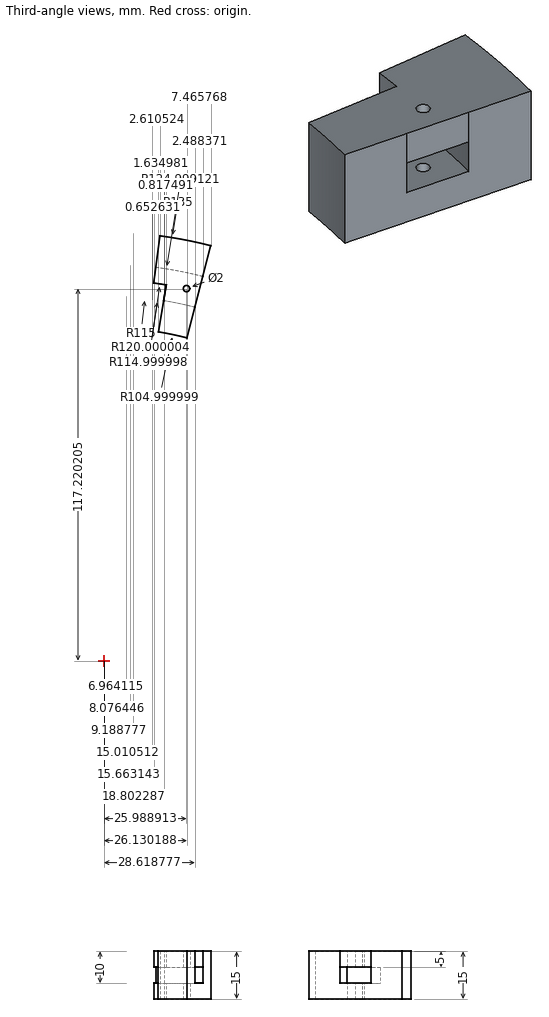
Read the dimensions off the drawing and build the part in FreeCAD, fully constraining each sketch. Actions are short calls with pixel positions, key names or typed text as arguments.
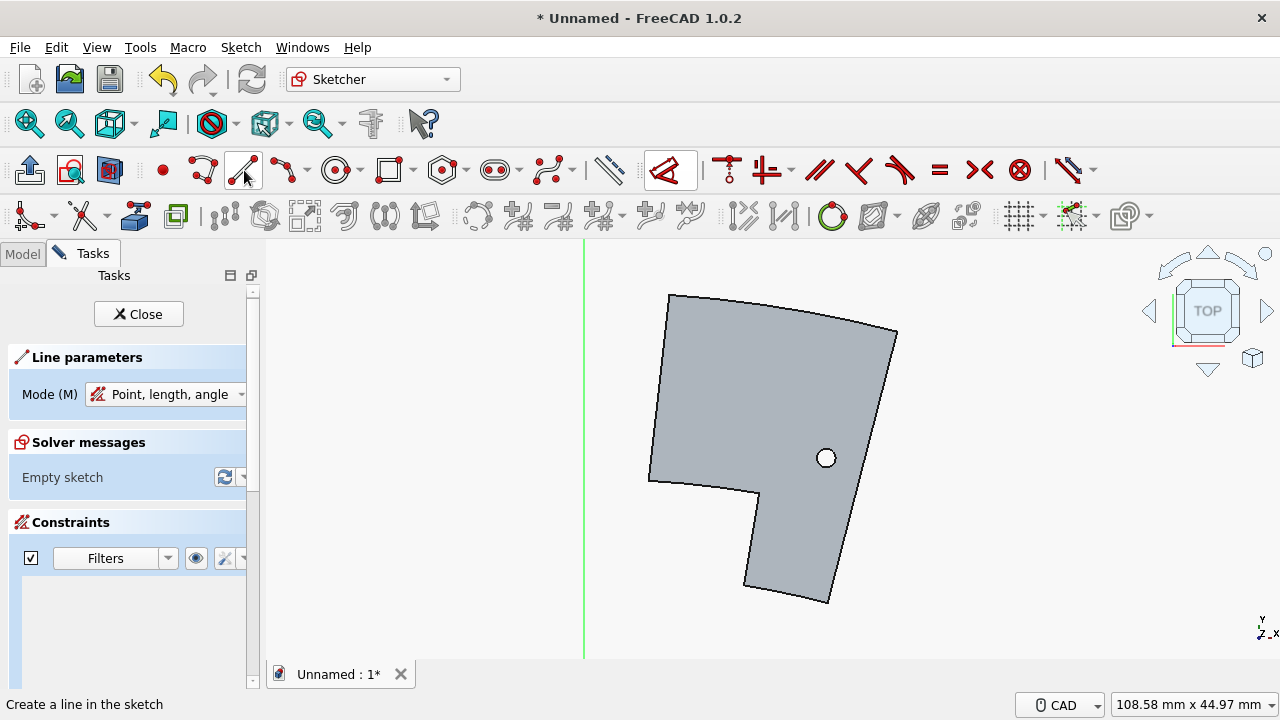
click(584, 292)
click(593, 479)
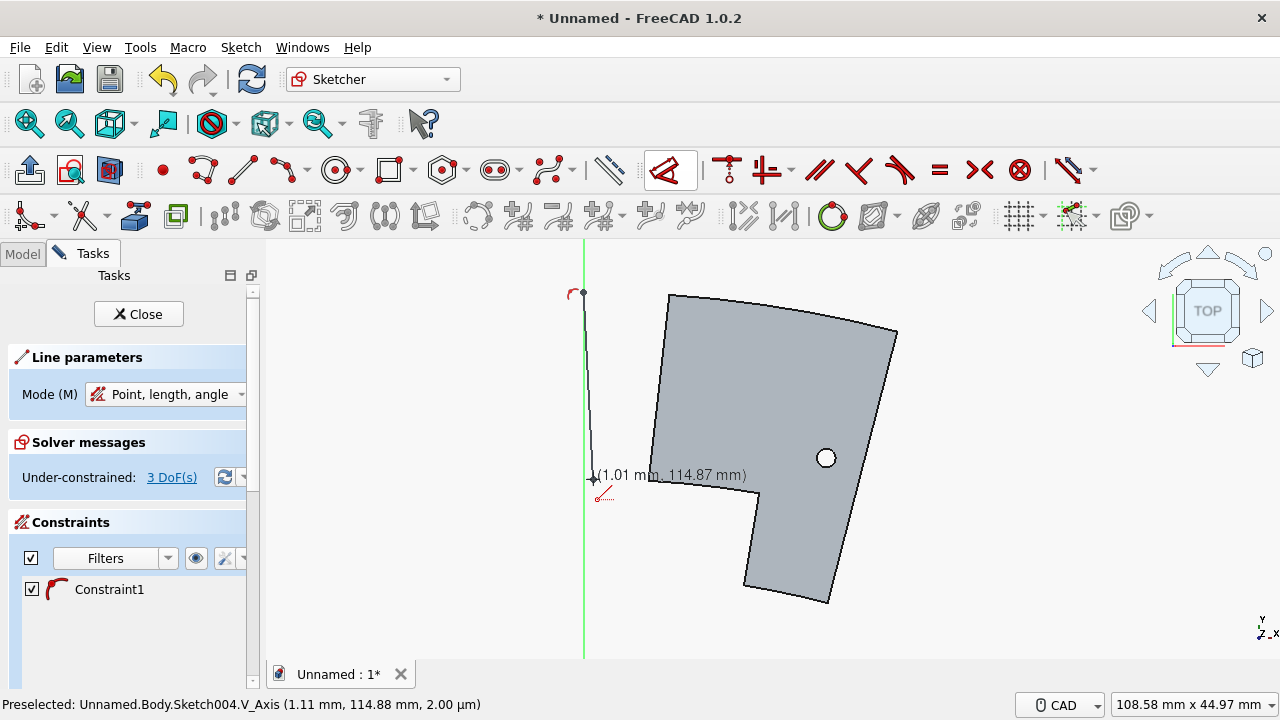
click(724, 488)
click(748, 303)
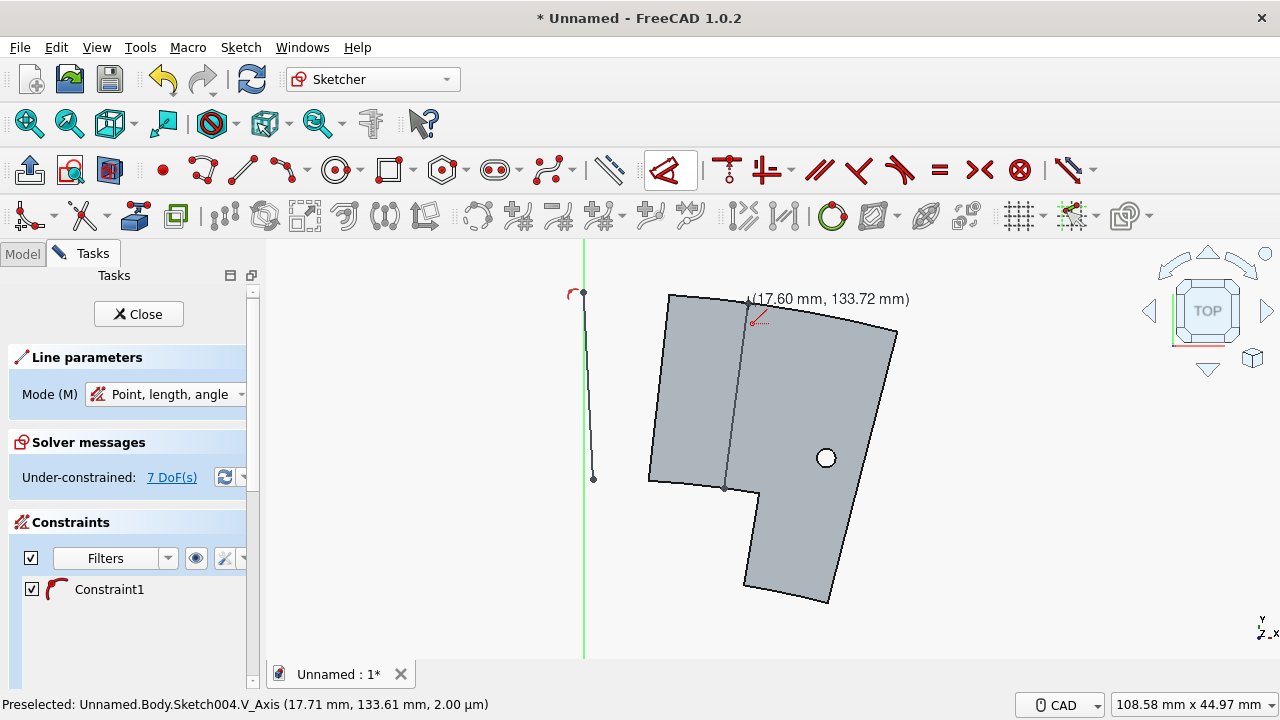
click(284, 170)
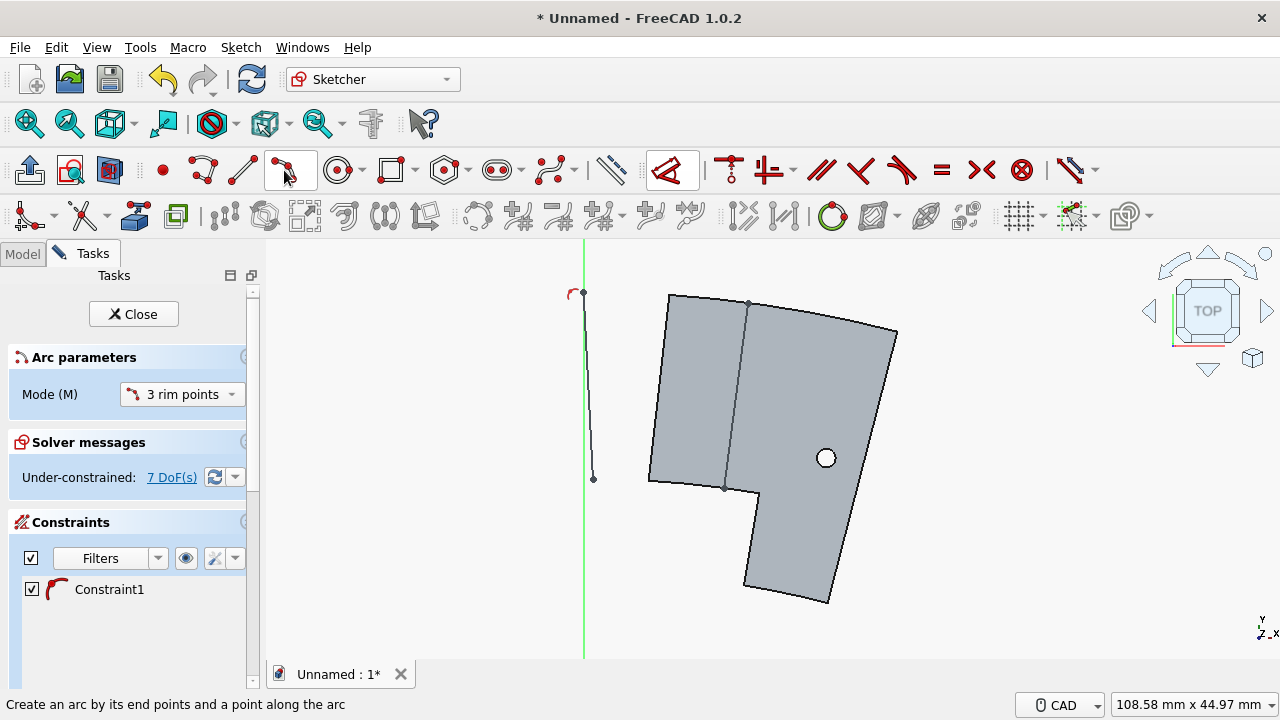
click(593, 480)
click(724, 489)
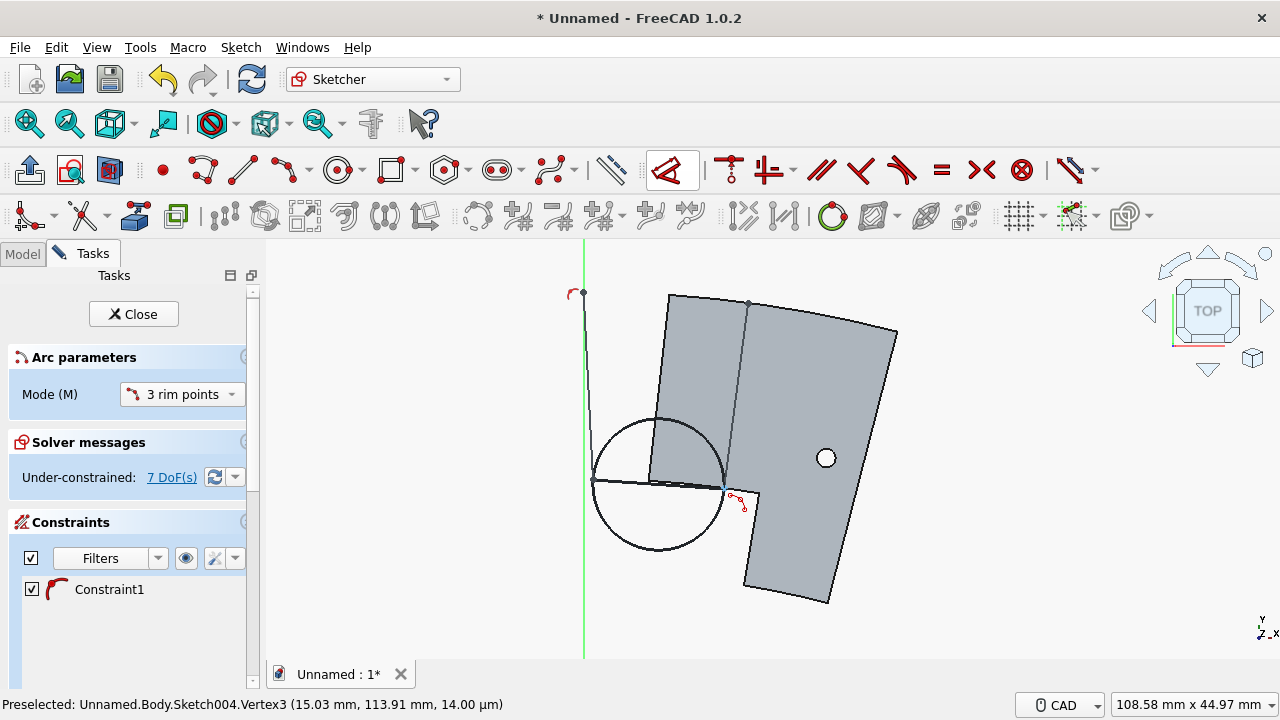
scroll(654, 481, up, 10)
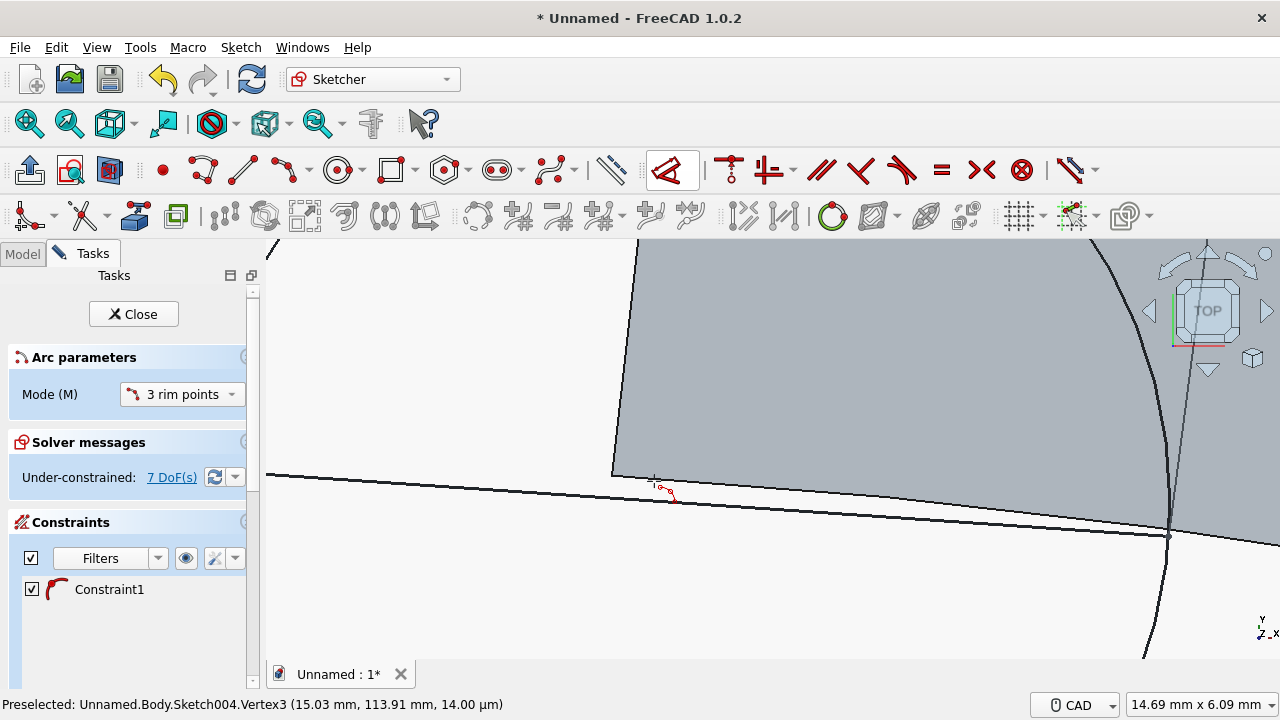
click(650, 478)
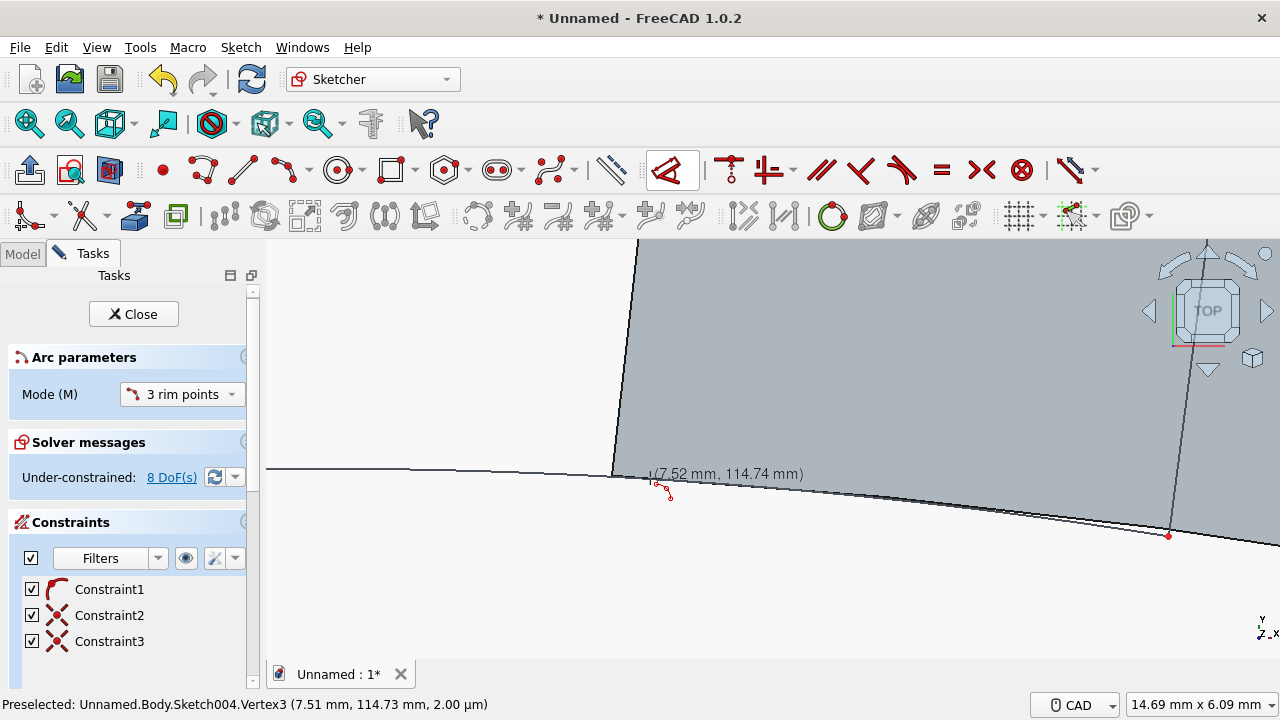
scroll(698, 577, down, 9)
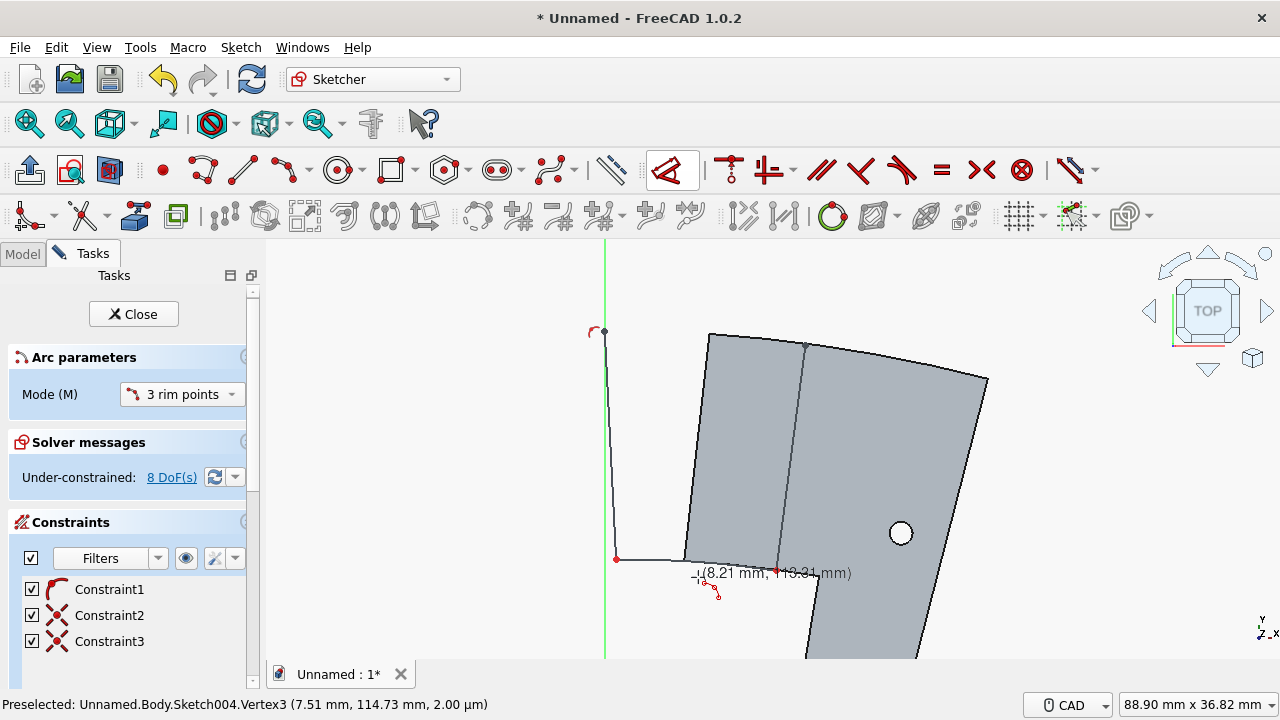
click(805, 345)
click(605, 332)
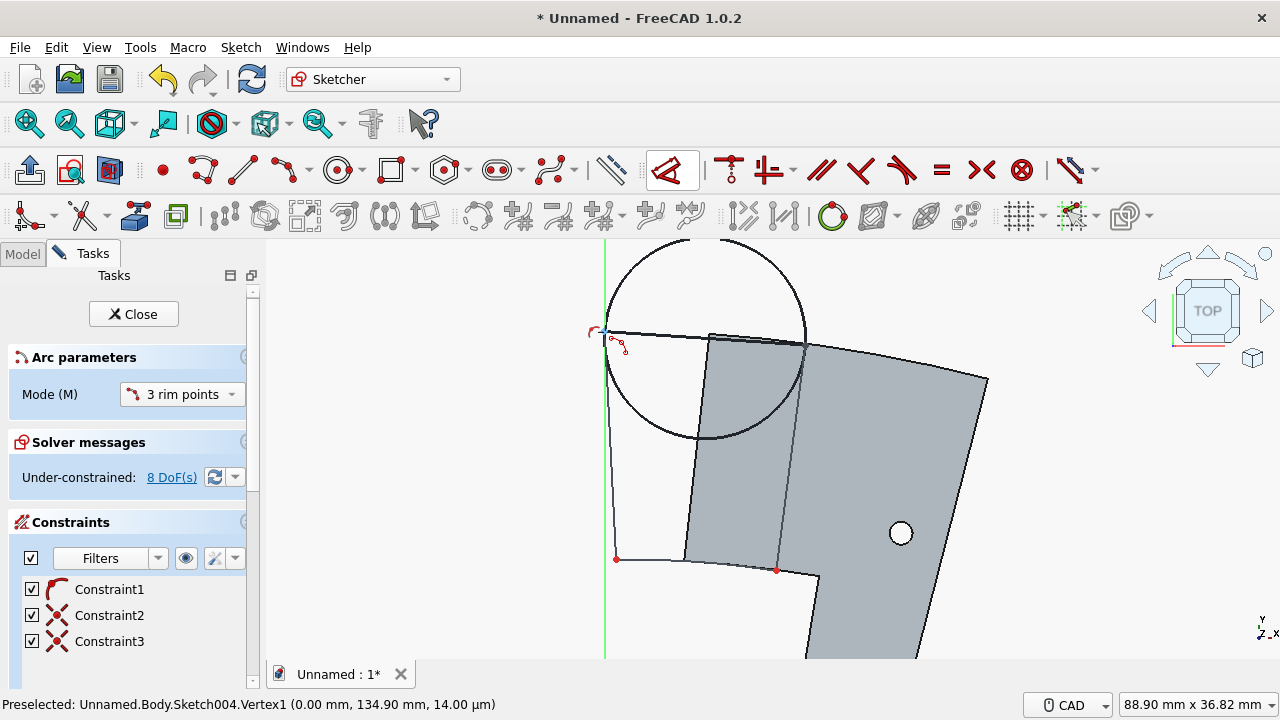
scroll(705, 334, up, 8)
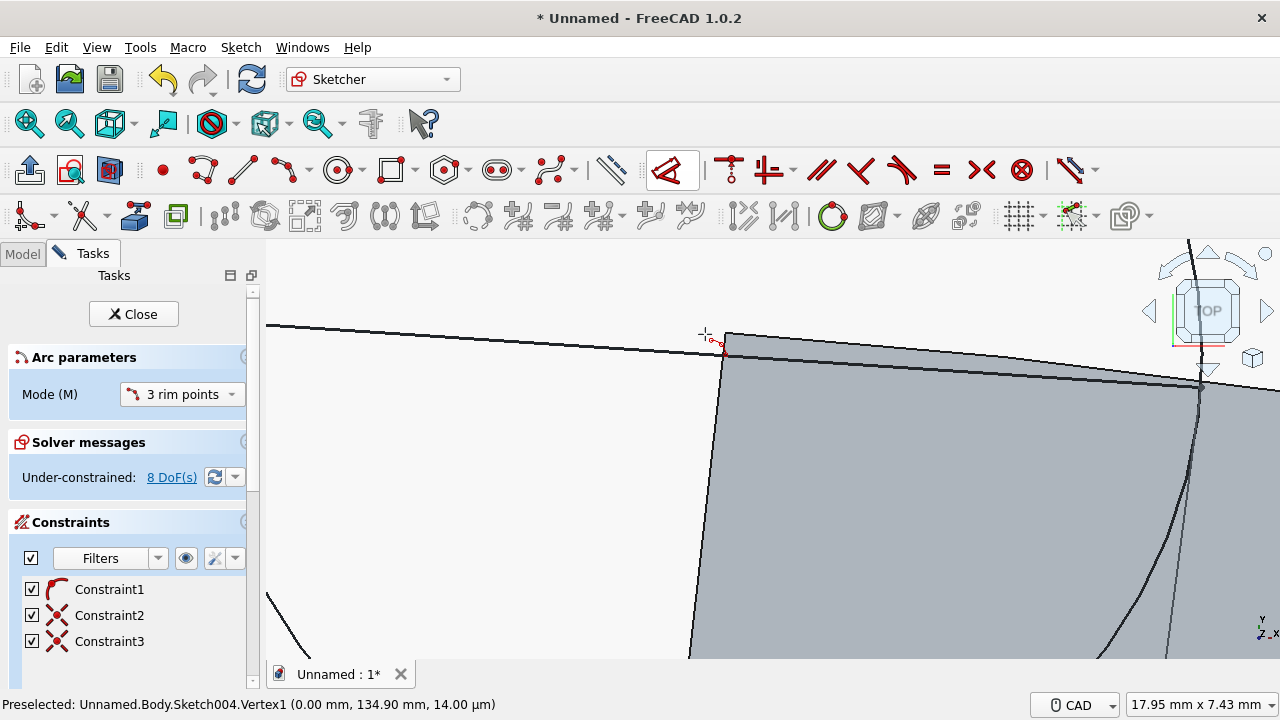
click(705, 332)
key(Escape)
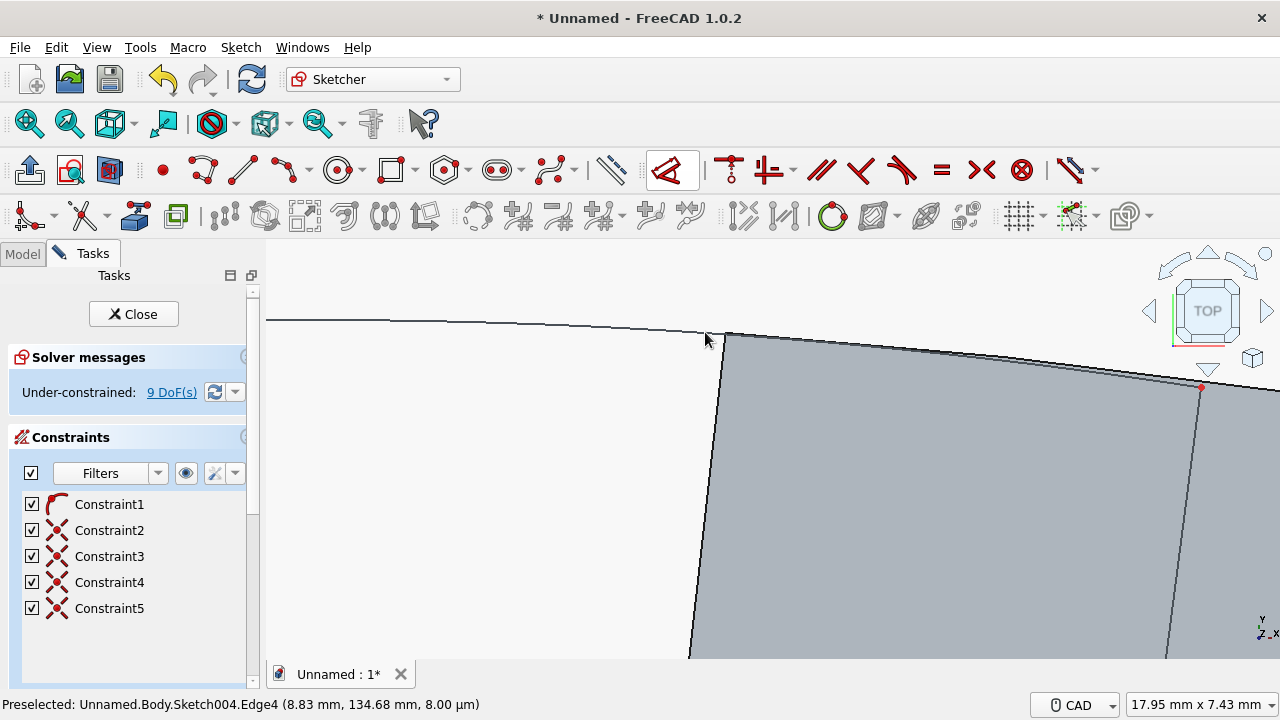
scroll(705, 333, down, 8)